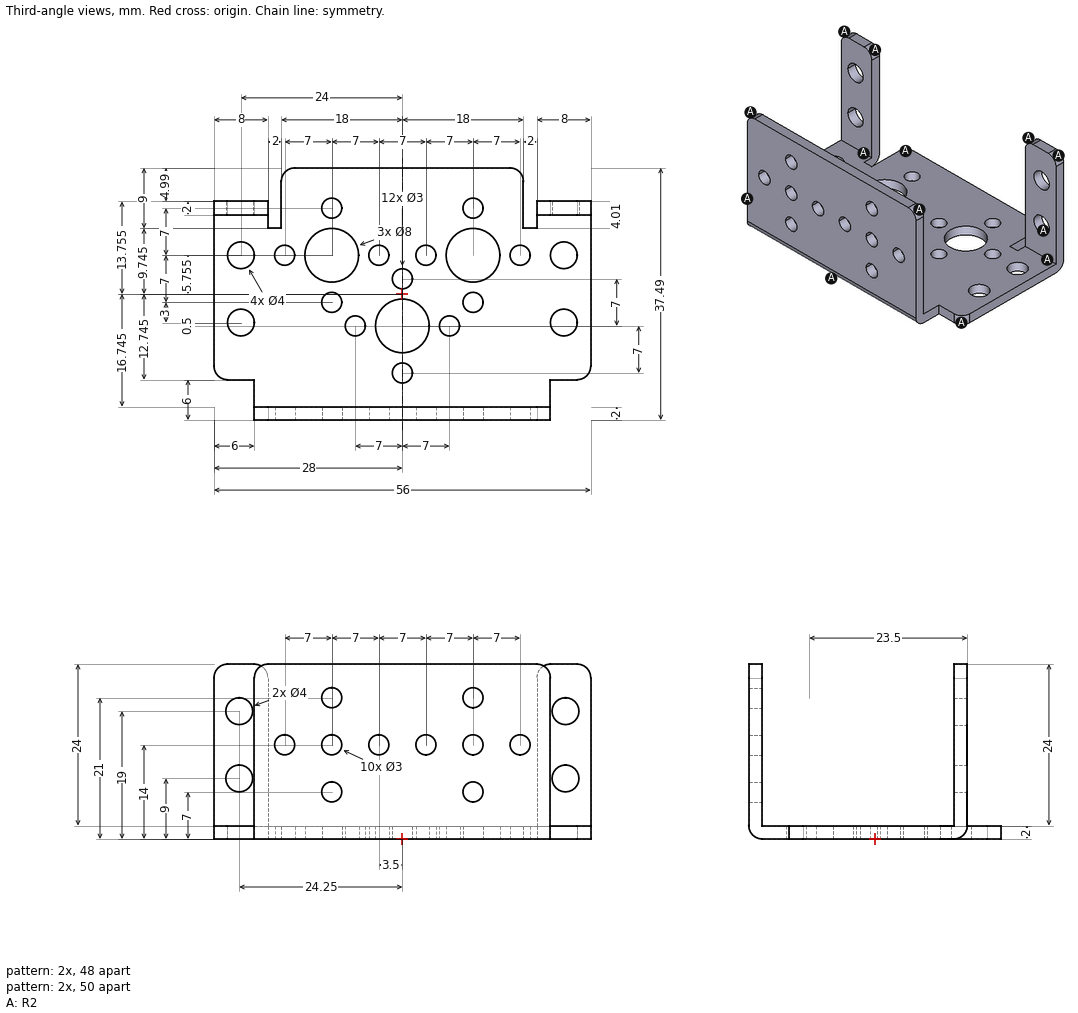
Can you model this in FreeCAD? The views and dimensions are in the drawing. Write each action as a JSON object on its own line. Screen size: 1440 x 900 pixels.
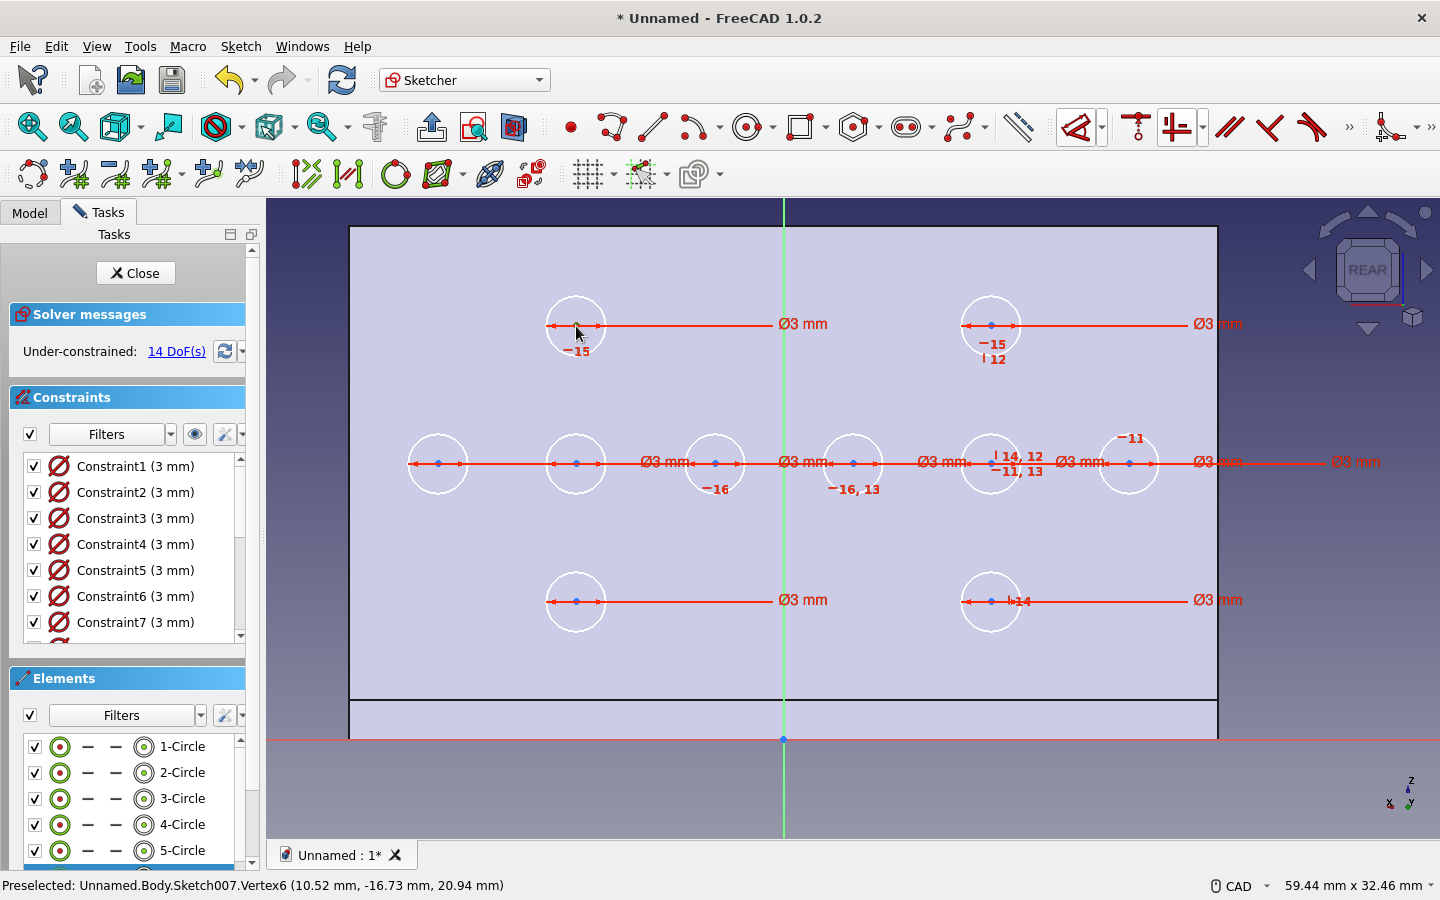
{"action": "left_click", "coordinate": [576, 602]}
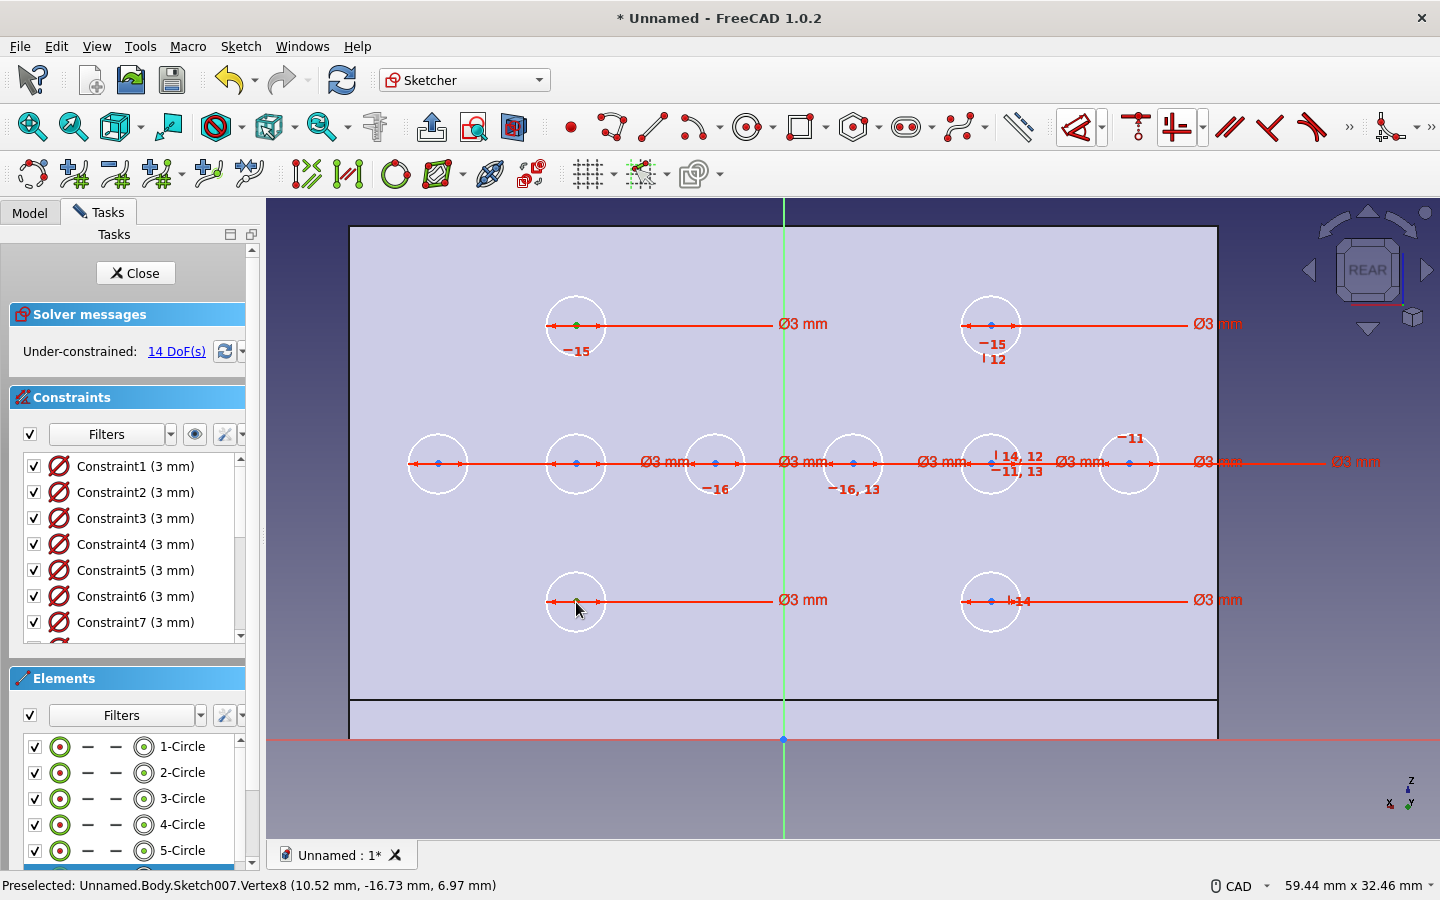
{"action": "key", "text": "v"}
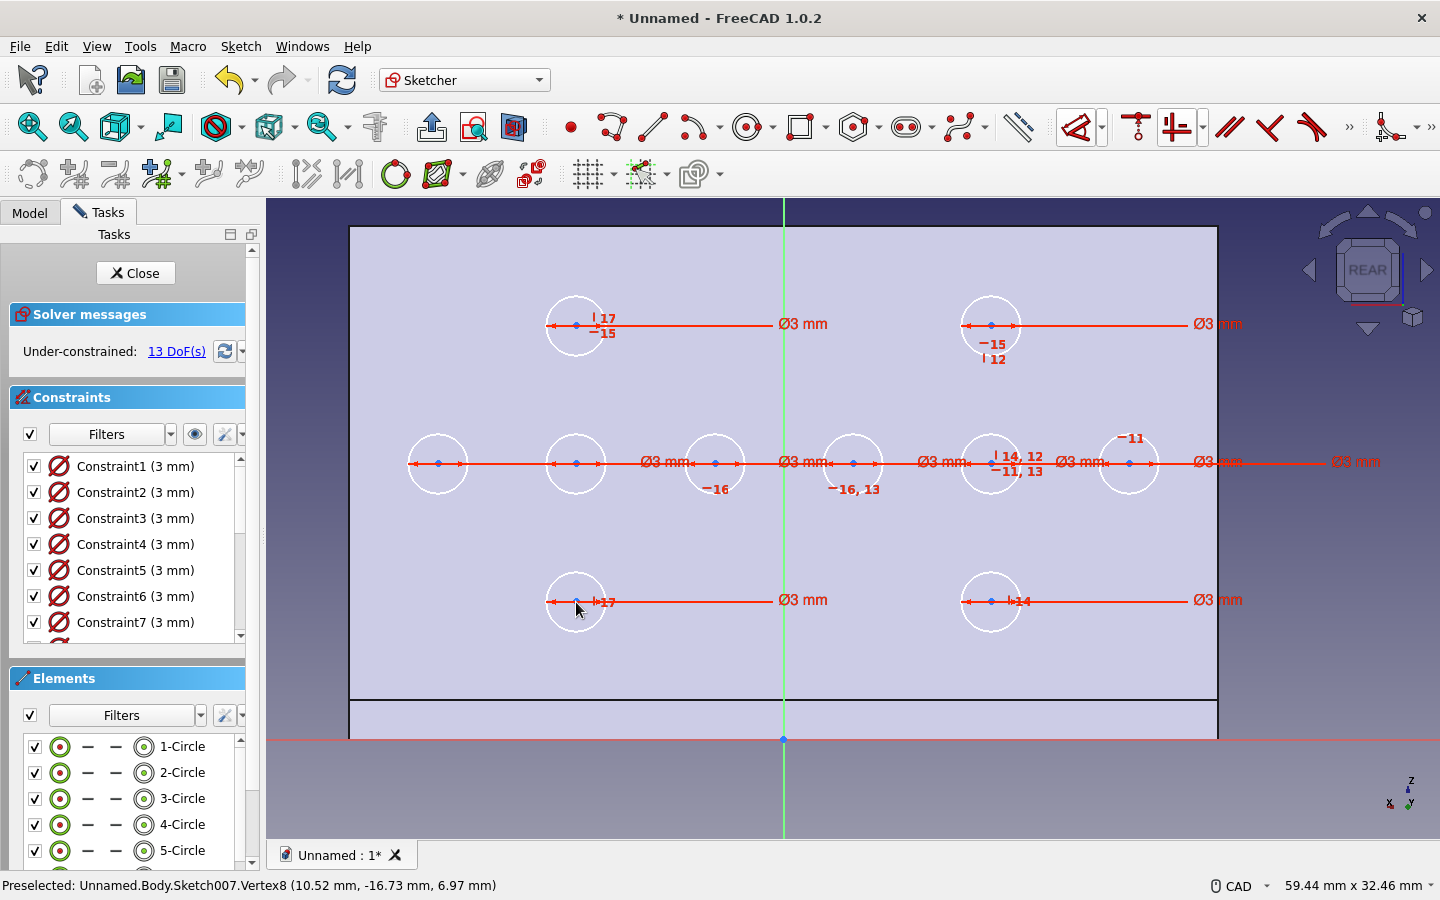
{"action": "left_click", "coordinate": [991, 602]}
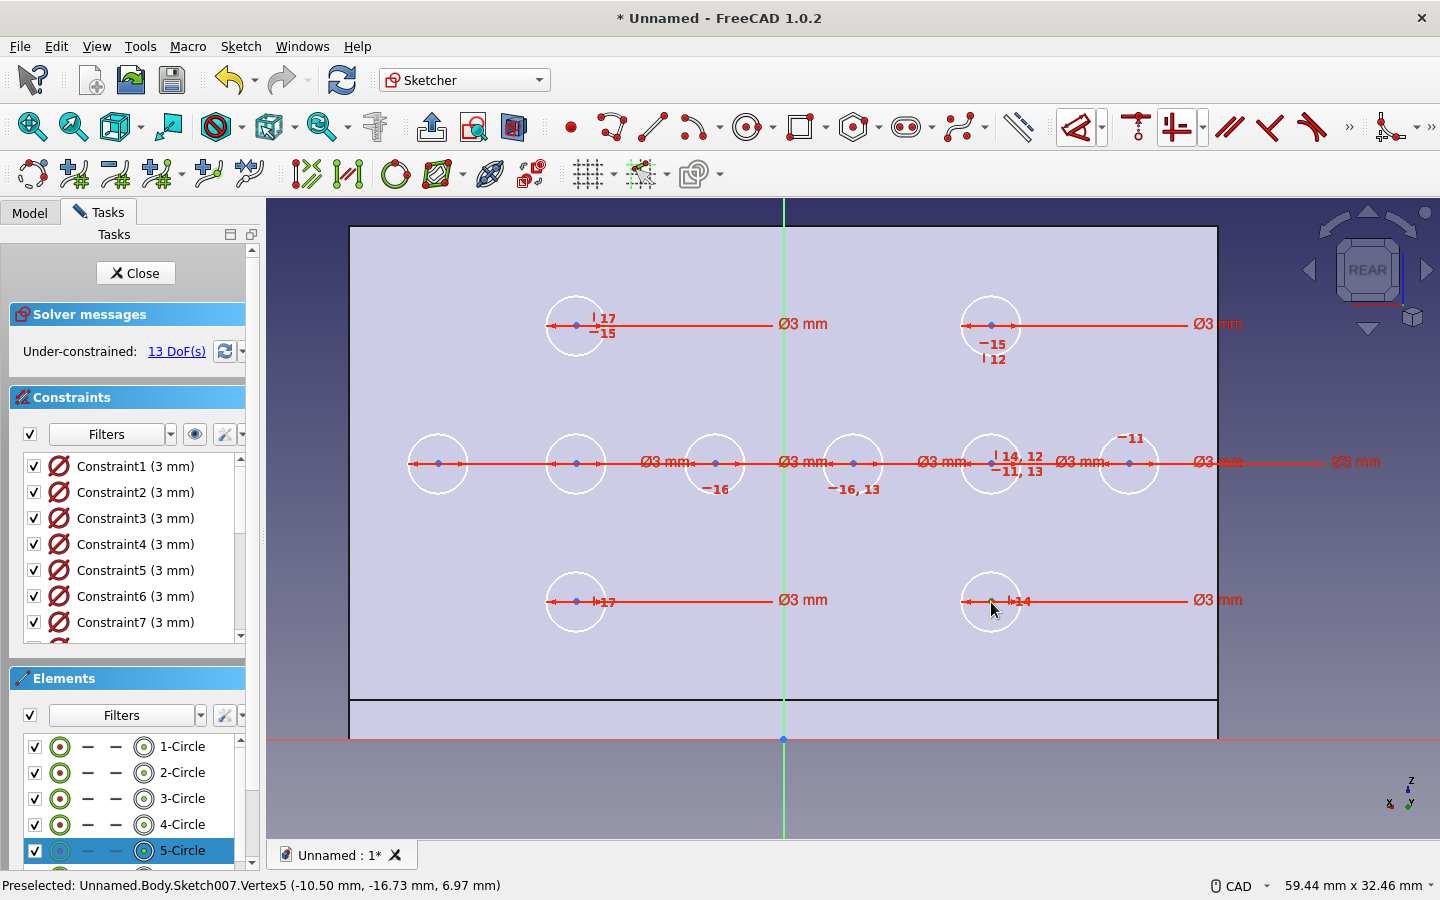
{"action": "left_click", "coordinate": [576, 602]}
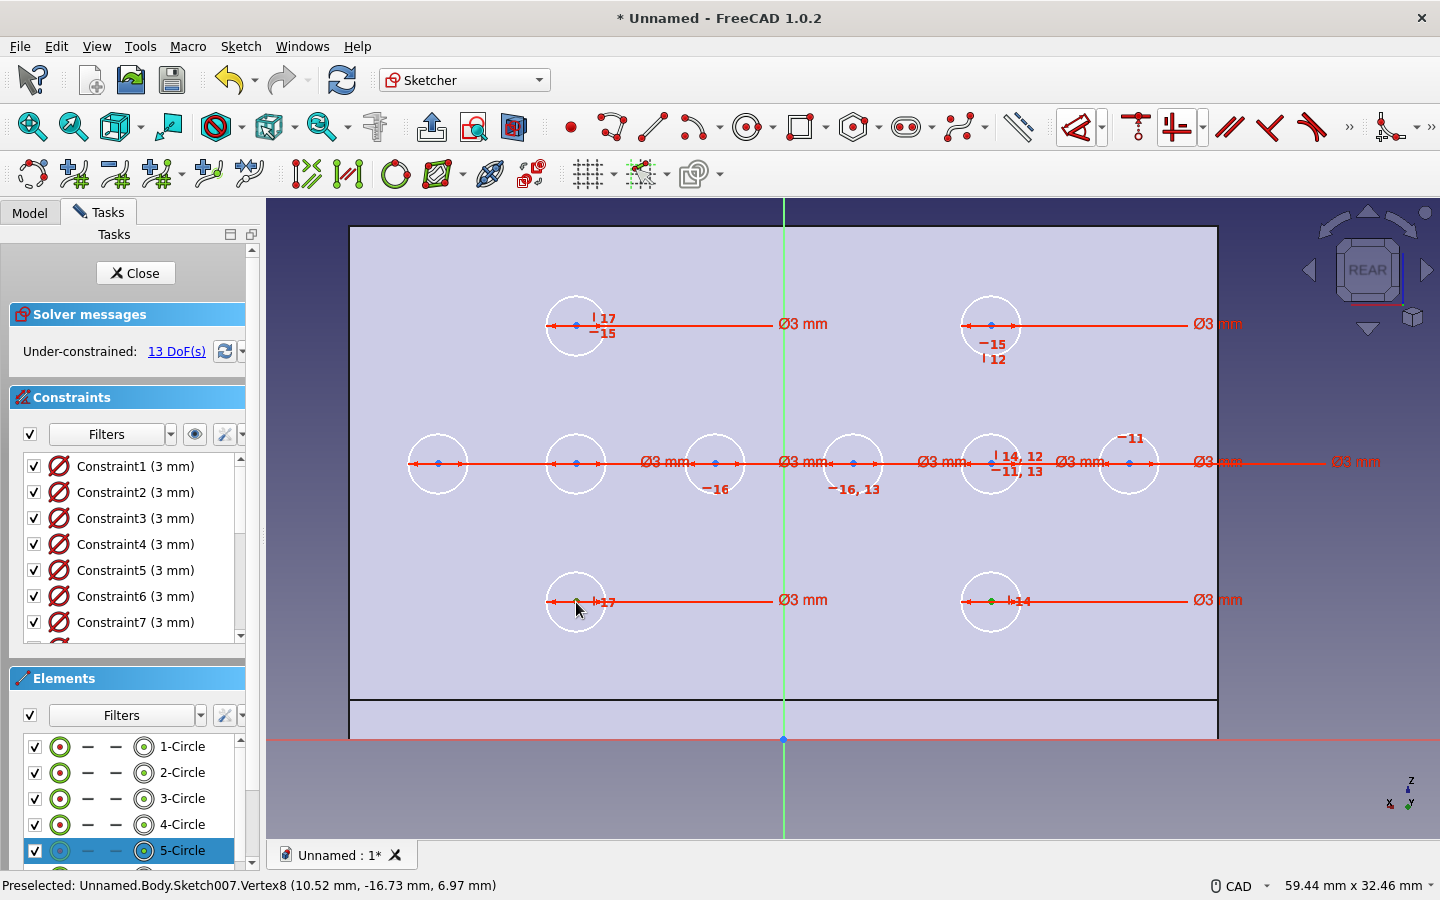
{"action": "key", "text": "h"}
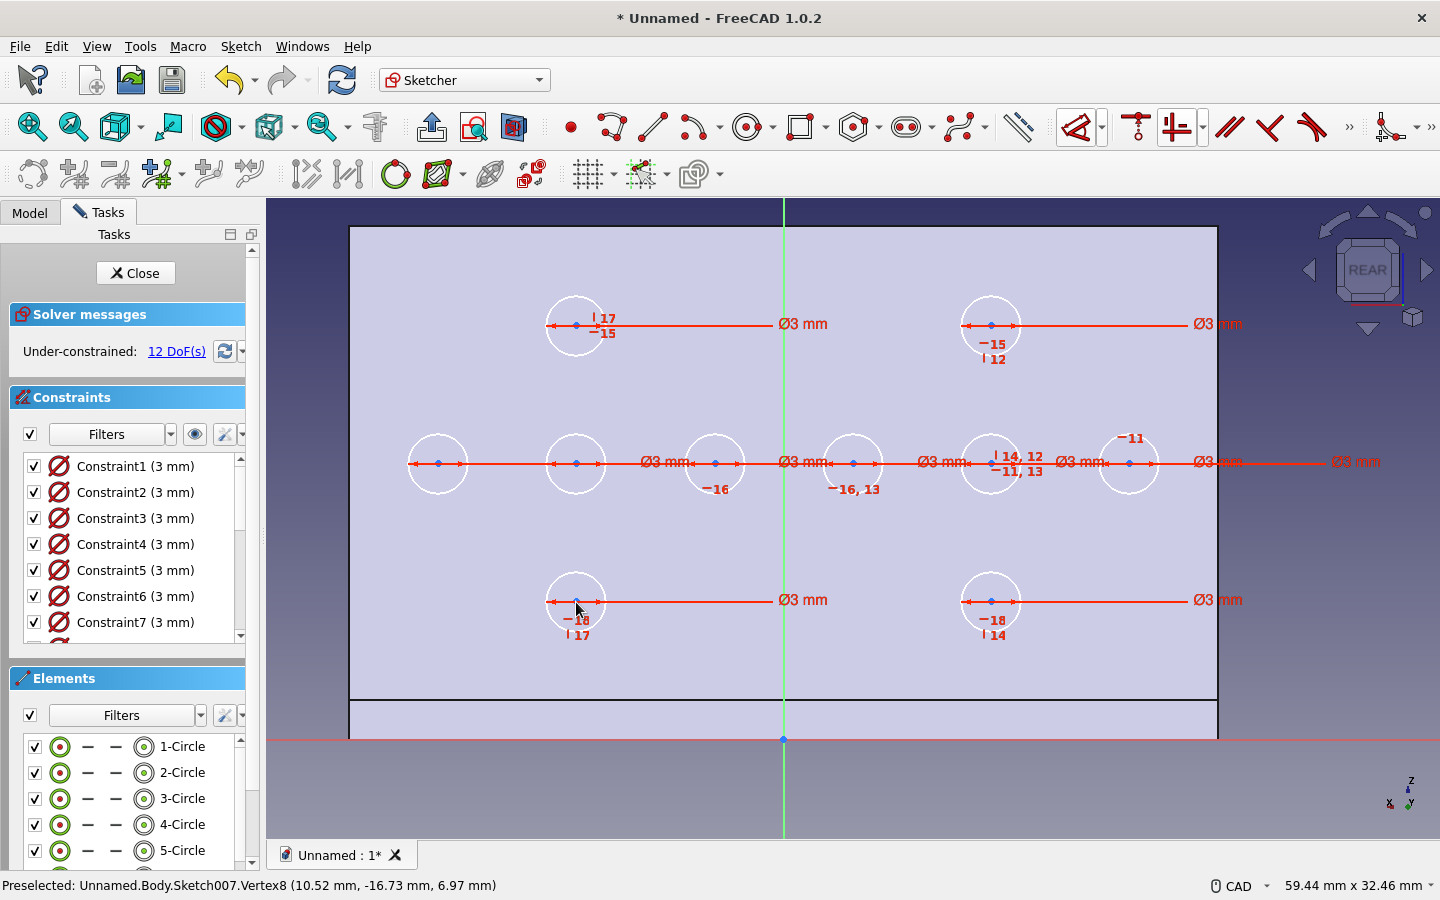
{"action": "left_click", "coordinate": [576, 326]}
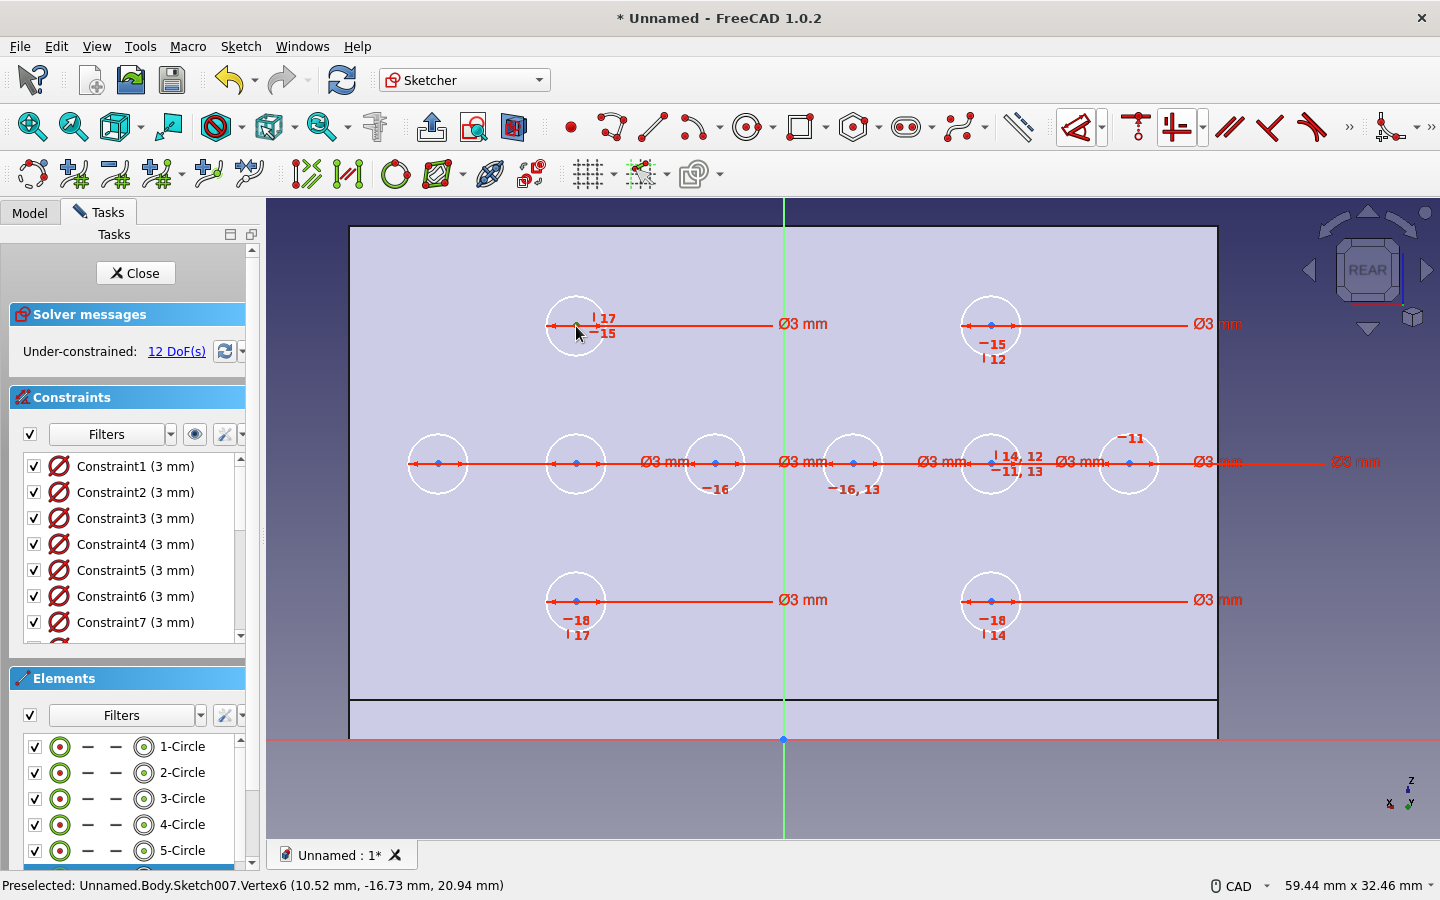
{"action": "left_click", "coordinate": [576, 464]}